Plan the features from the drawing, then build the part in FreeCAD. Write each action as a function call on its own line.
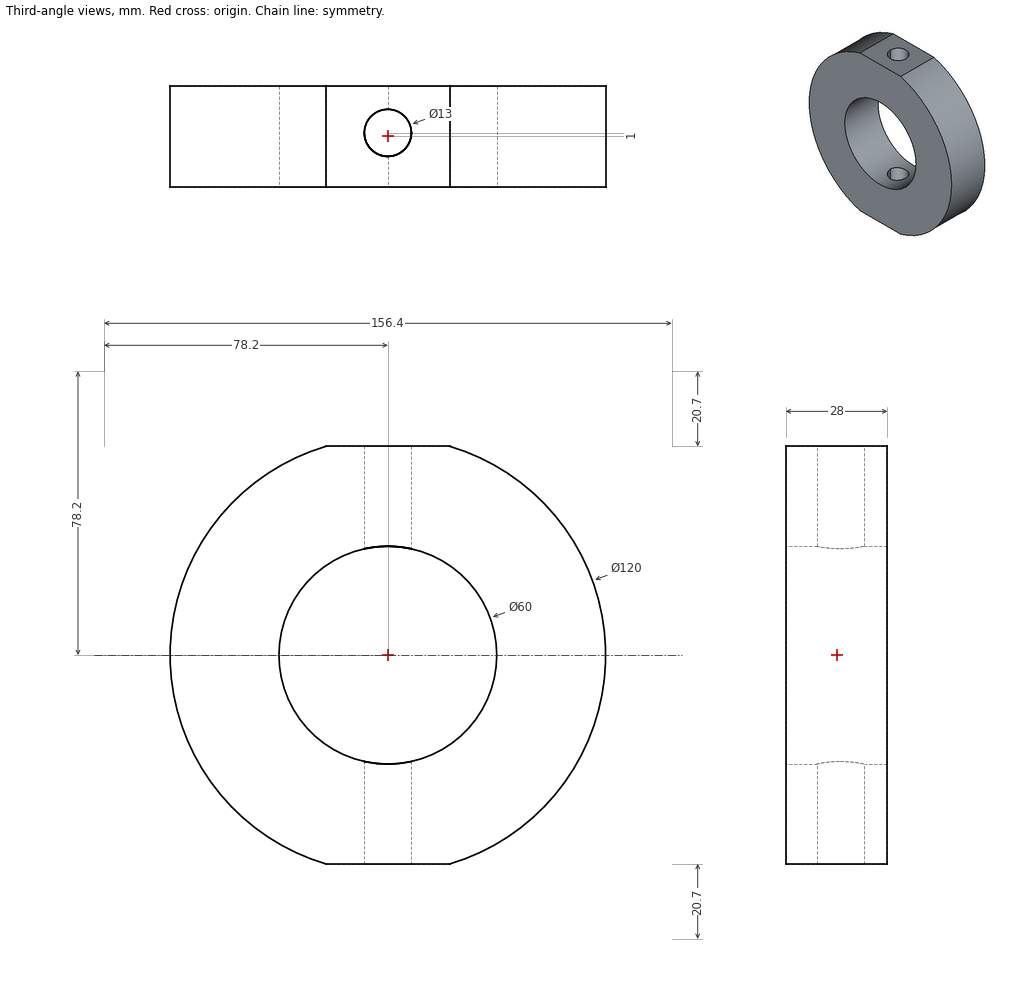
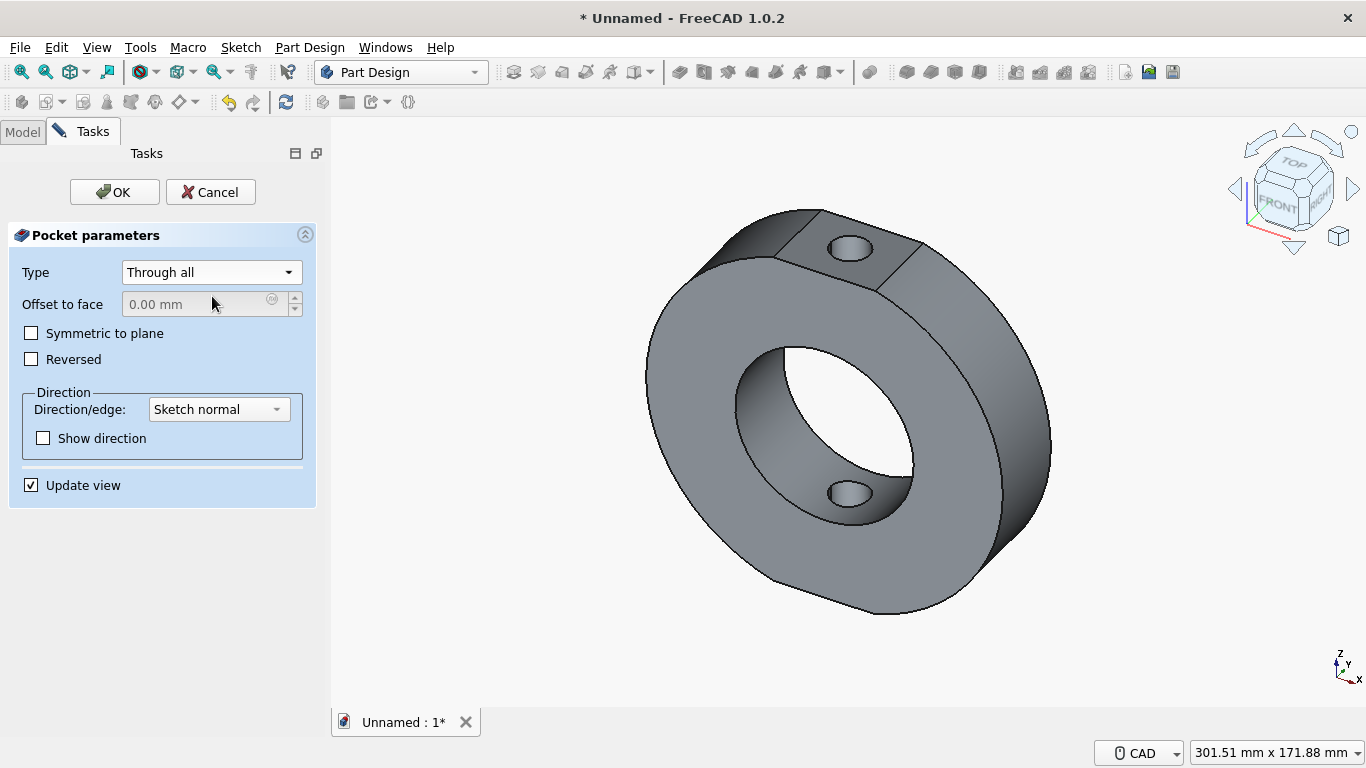
click(115, 192)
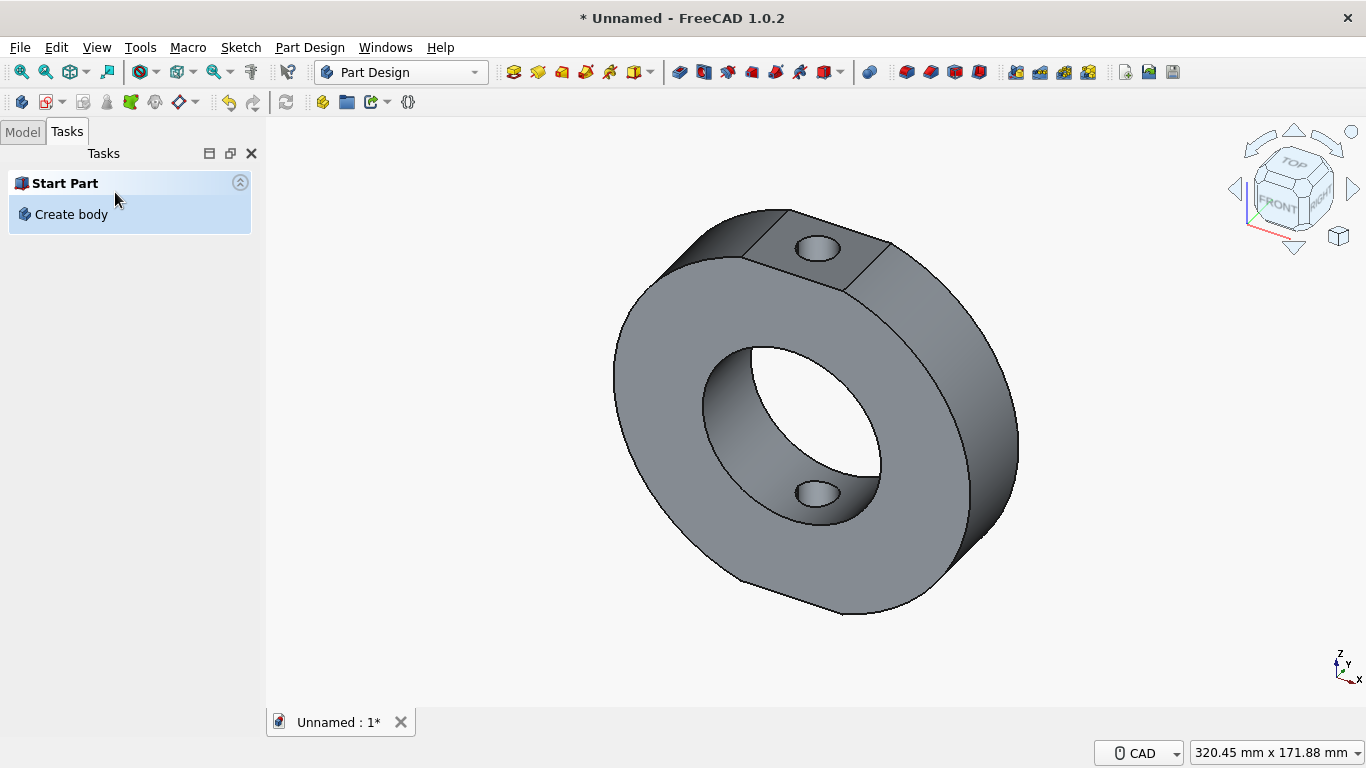
key(0)